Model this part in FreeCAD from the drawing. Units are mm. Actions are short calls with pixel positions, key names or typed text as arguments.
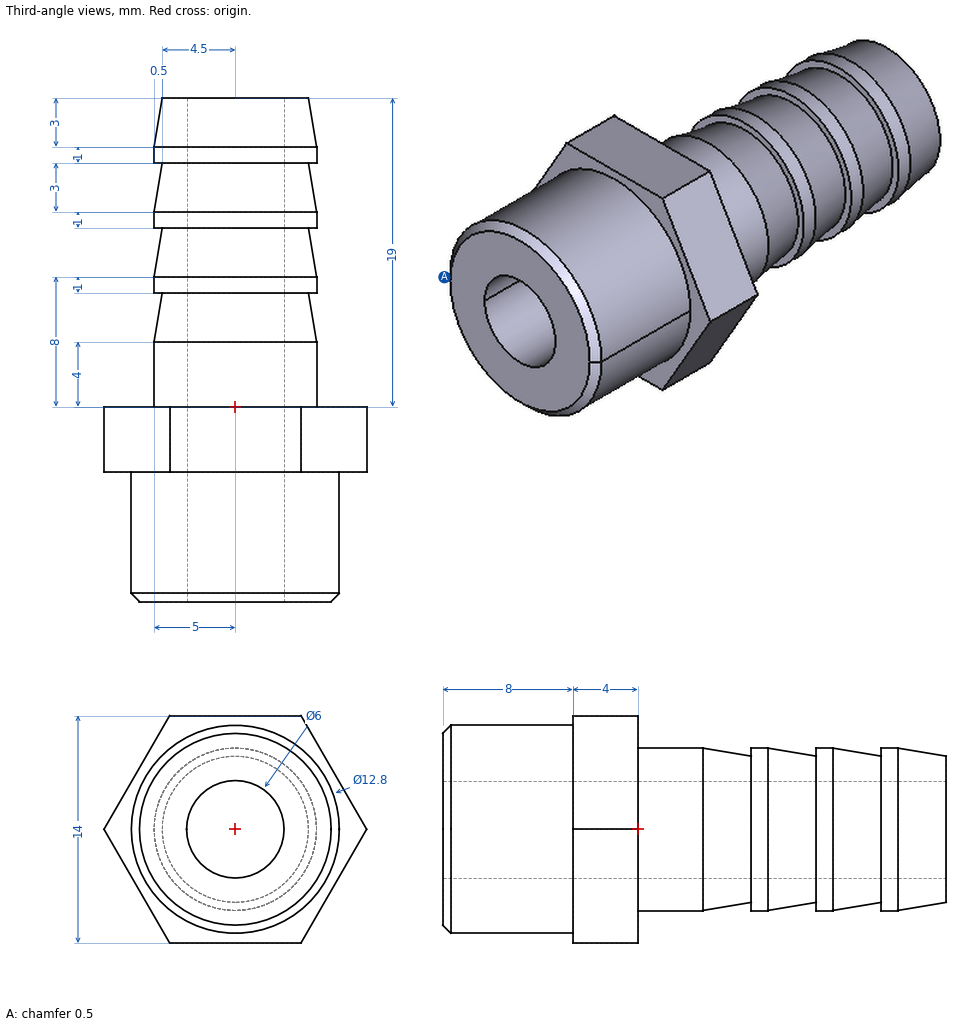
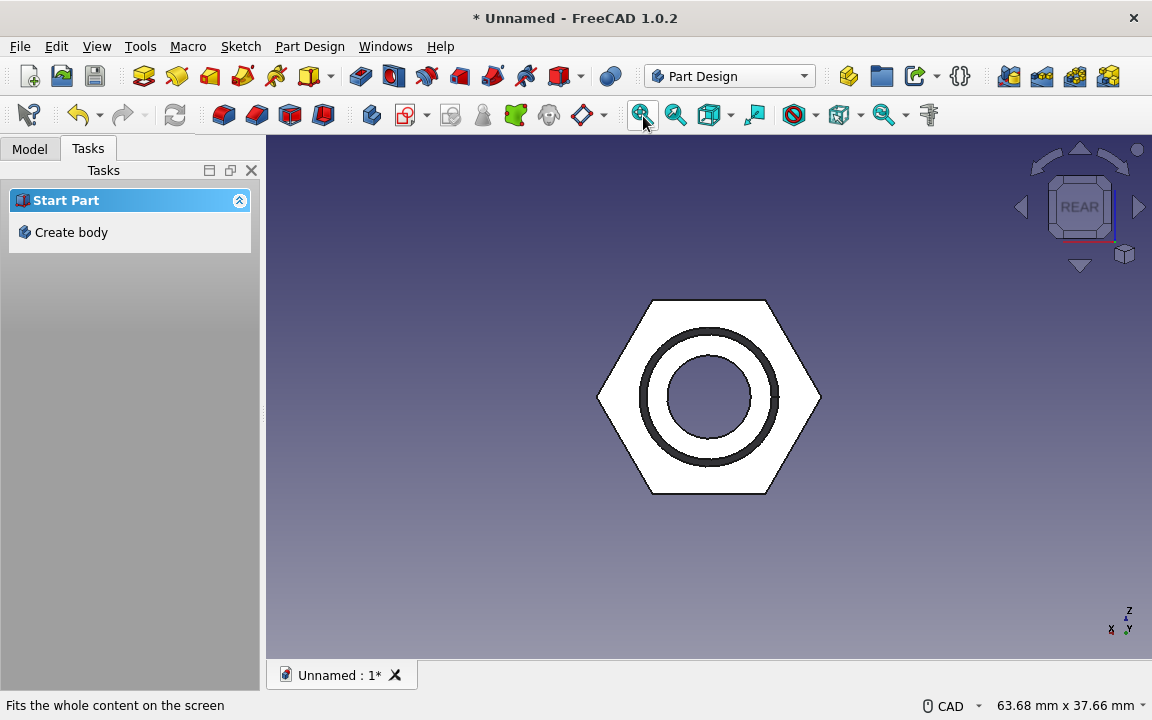
key(0)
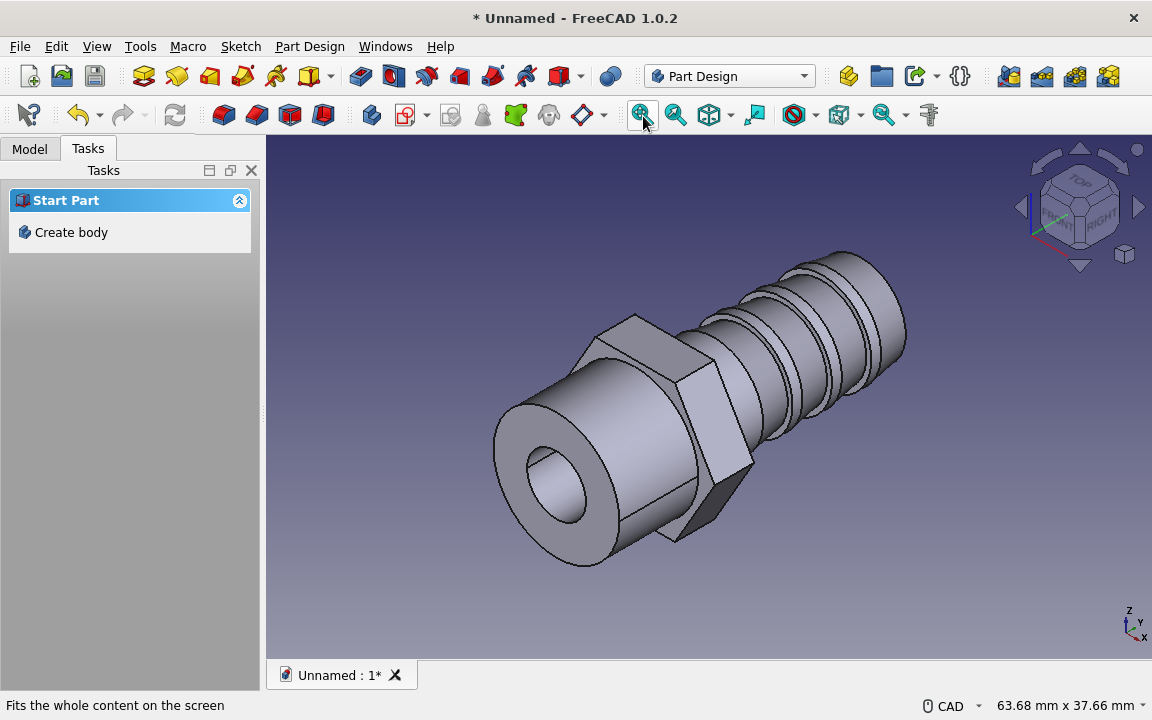
click(537, 404)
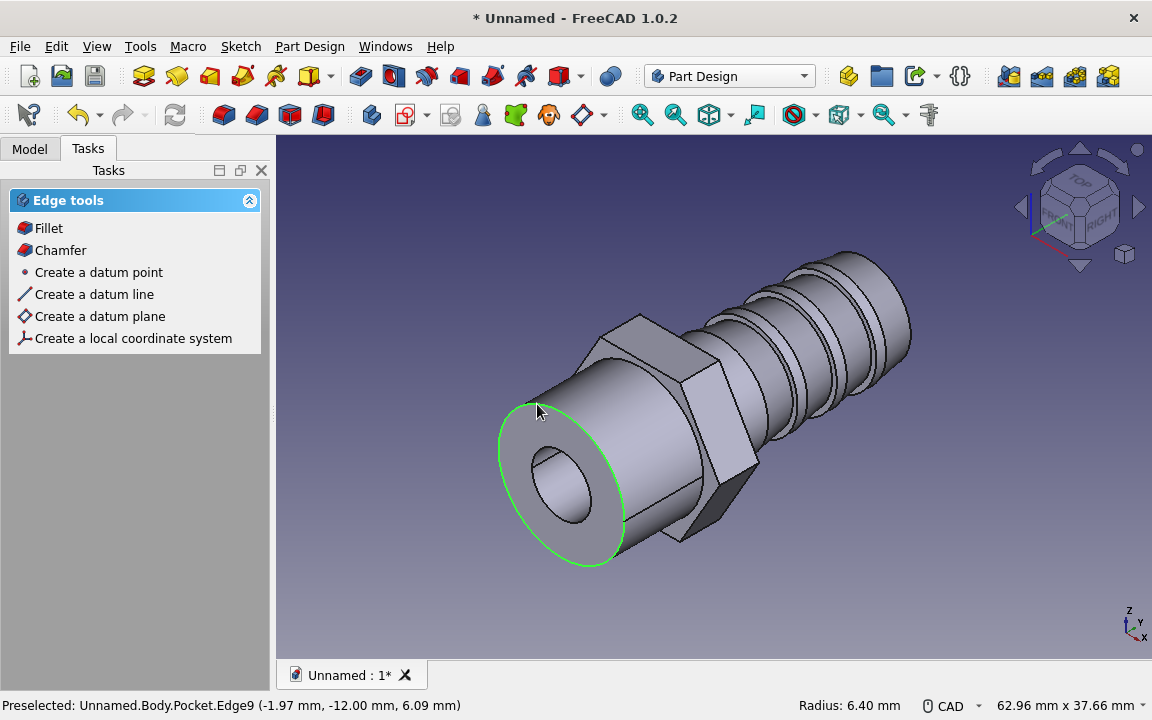
click(257, 116)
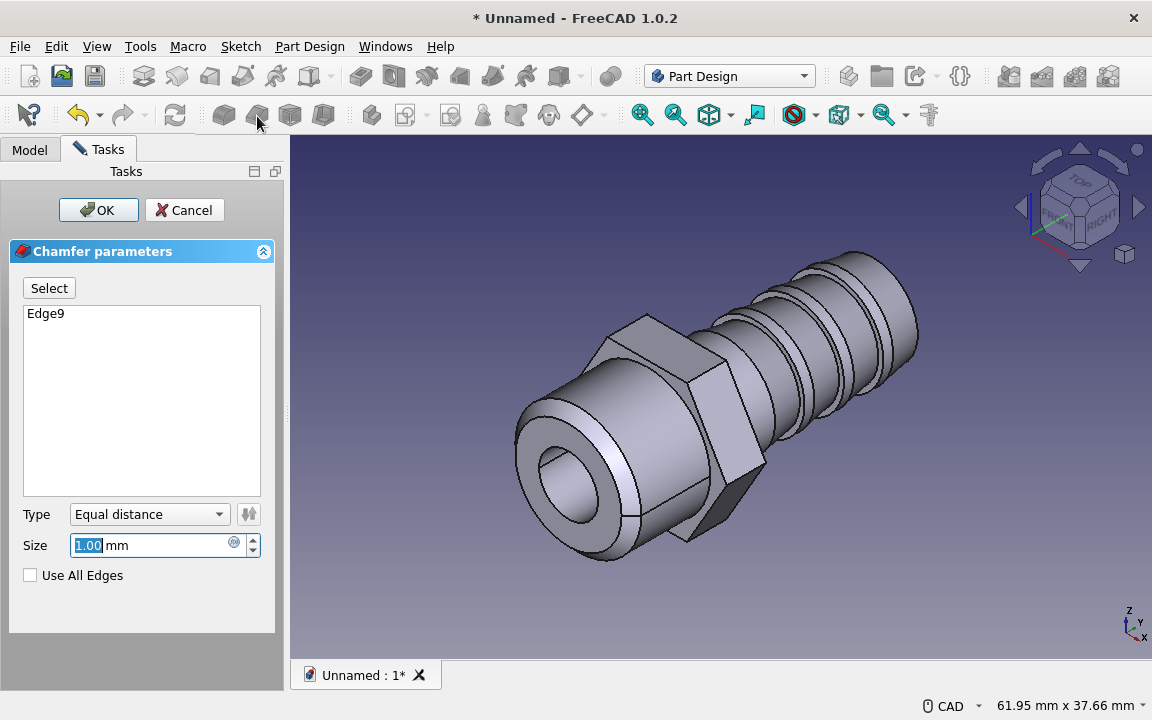
text(0.5)
key(Tab)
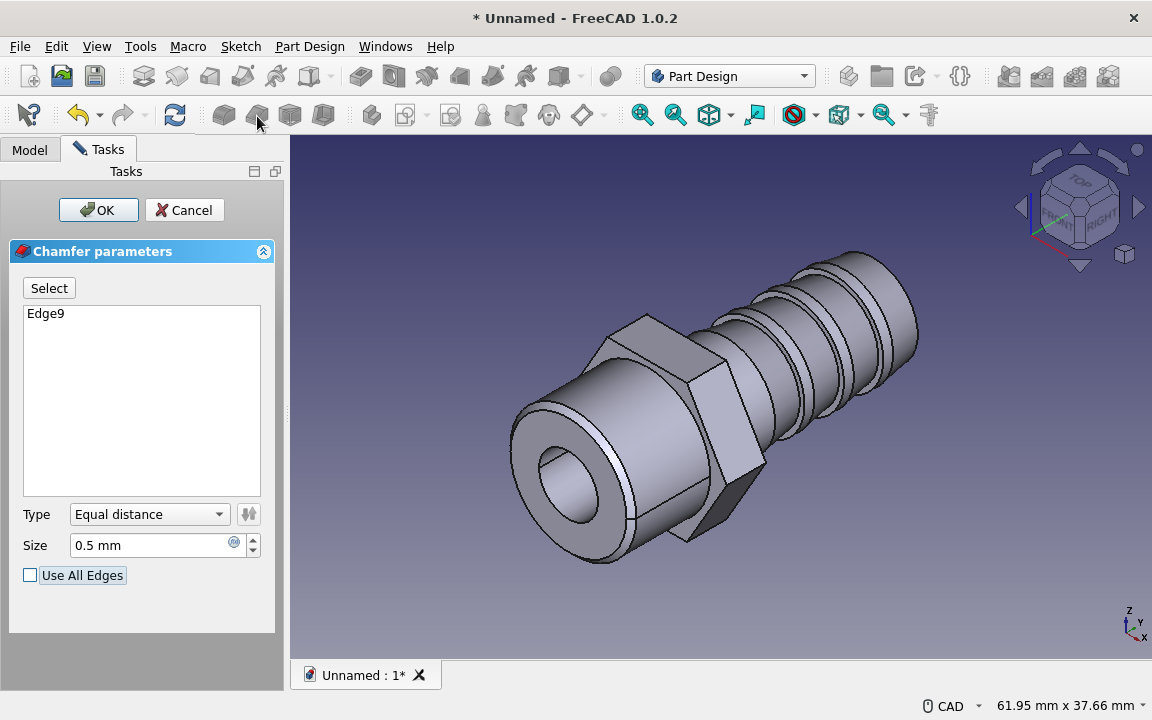
click(99, 210)